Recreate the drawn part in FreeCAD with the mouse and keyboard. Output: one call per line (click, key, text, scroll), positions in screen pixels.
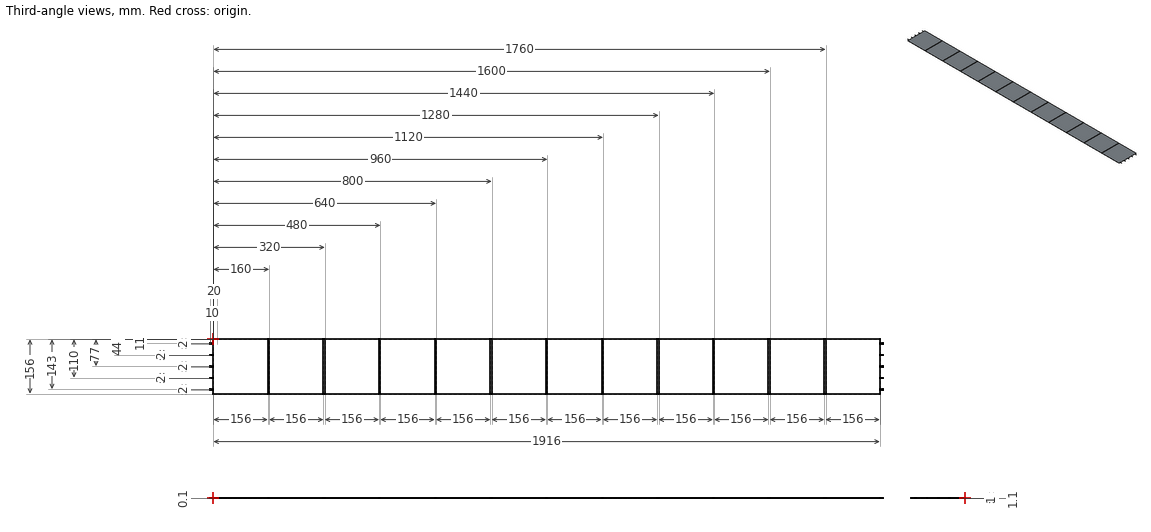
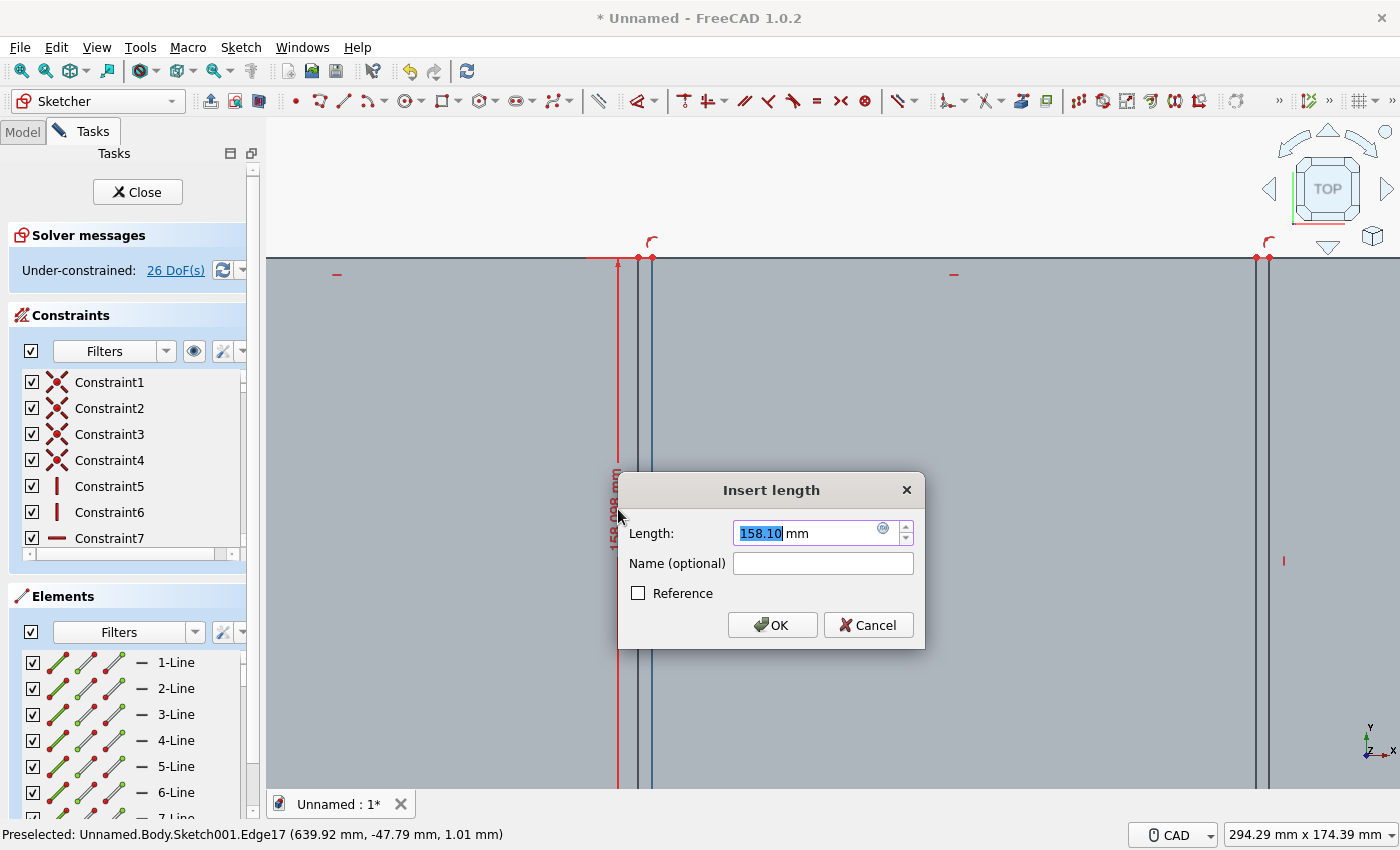
text(156)
key(Return)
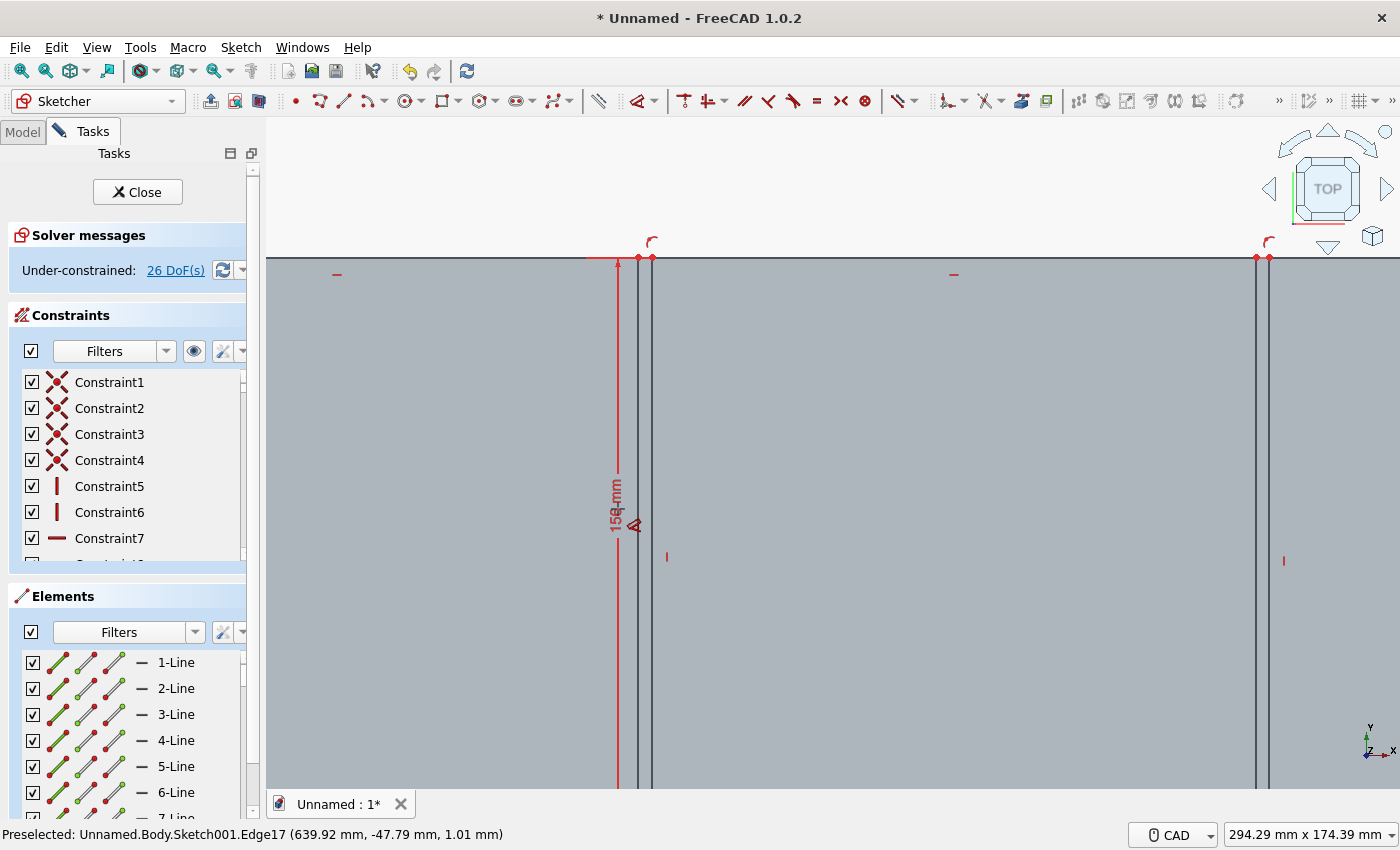
scroll(653, 442, down, 12)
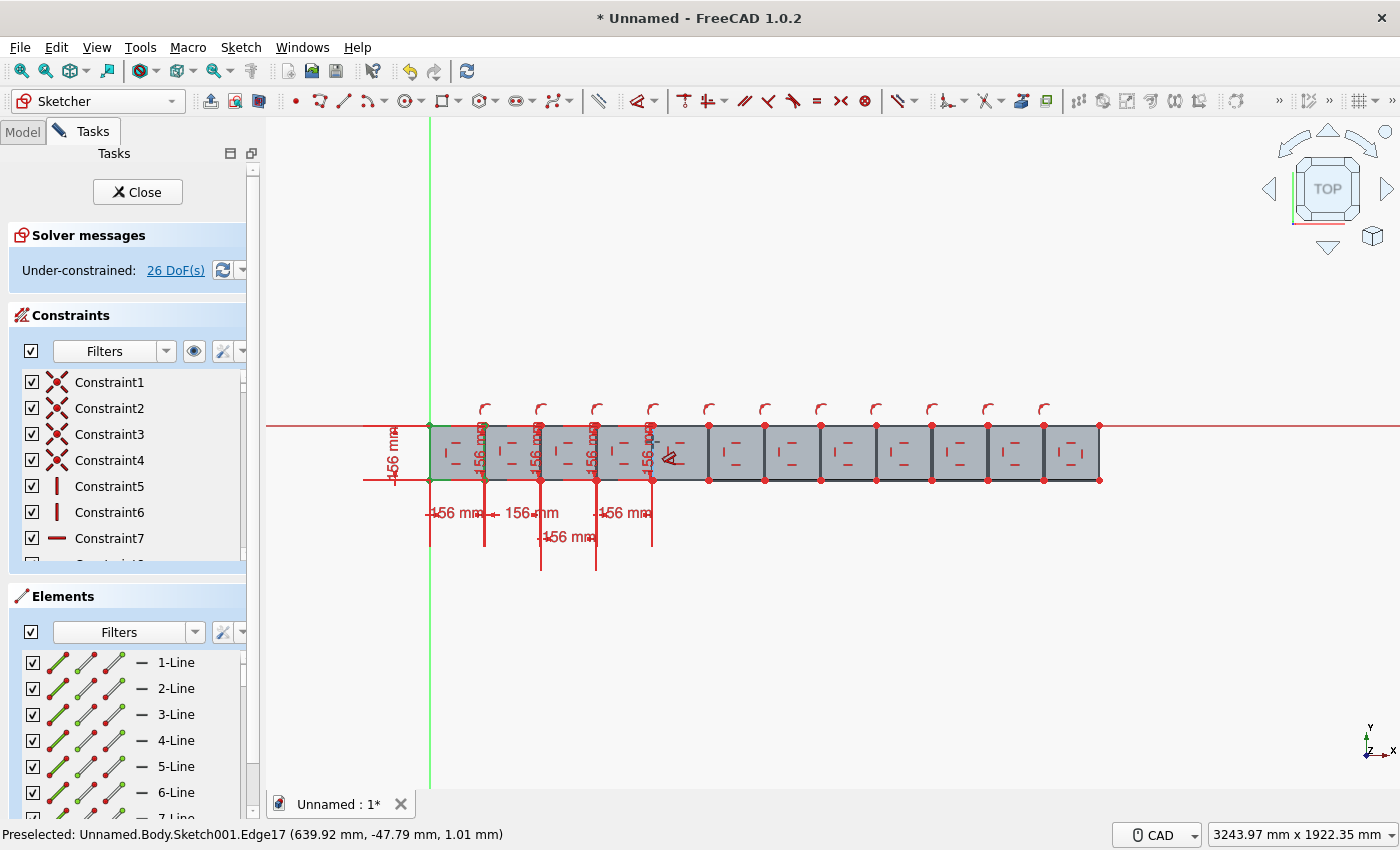
click(670, 480)
click(700, 514)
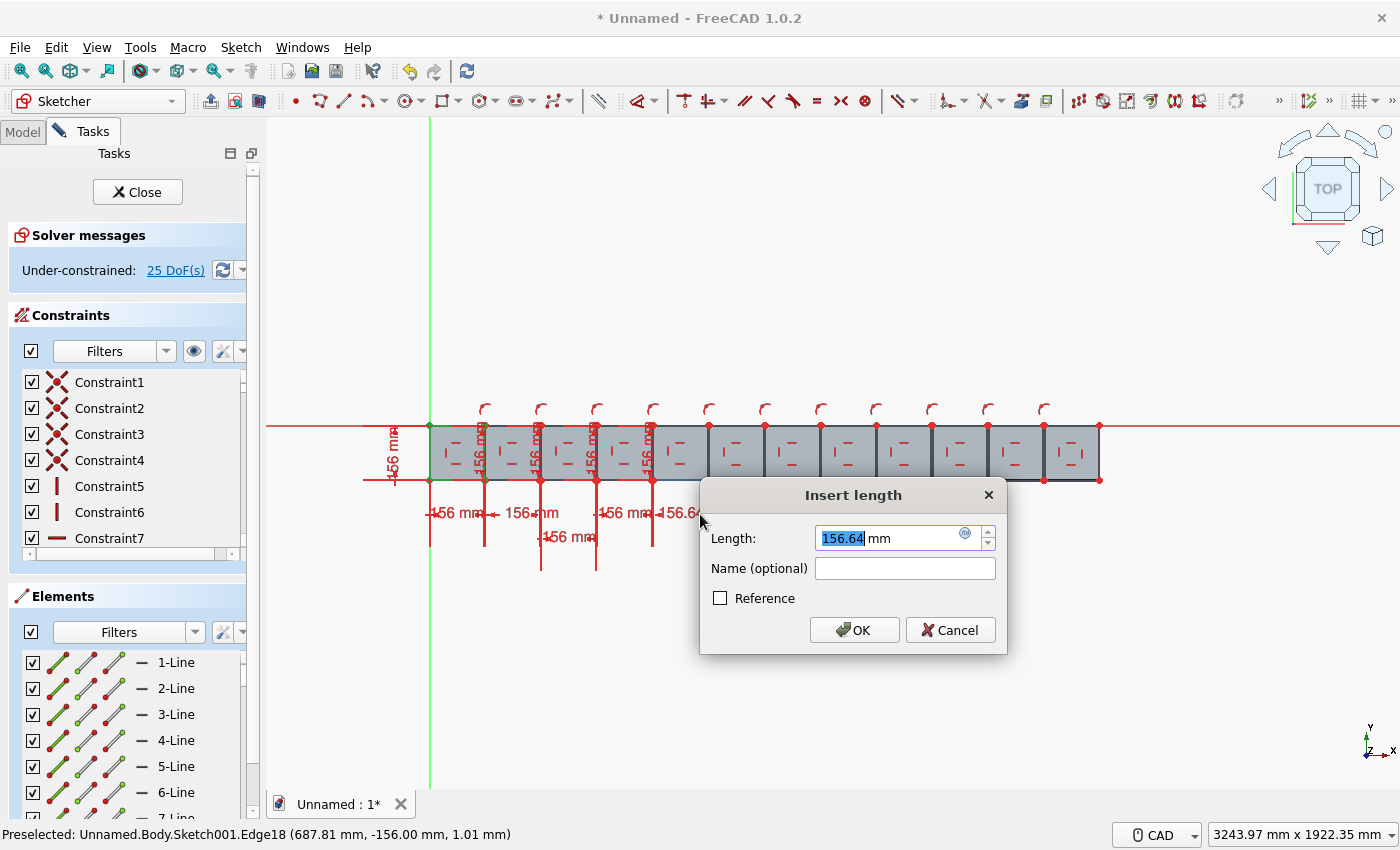
text(156)
key(Return)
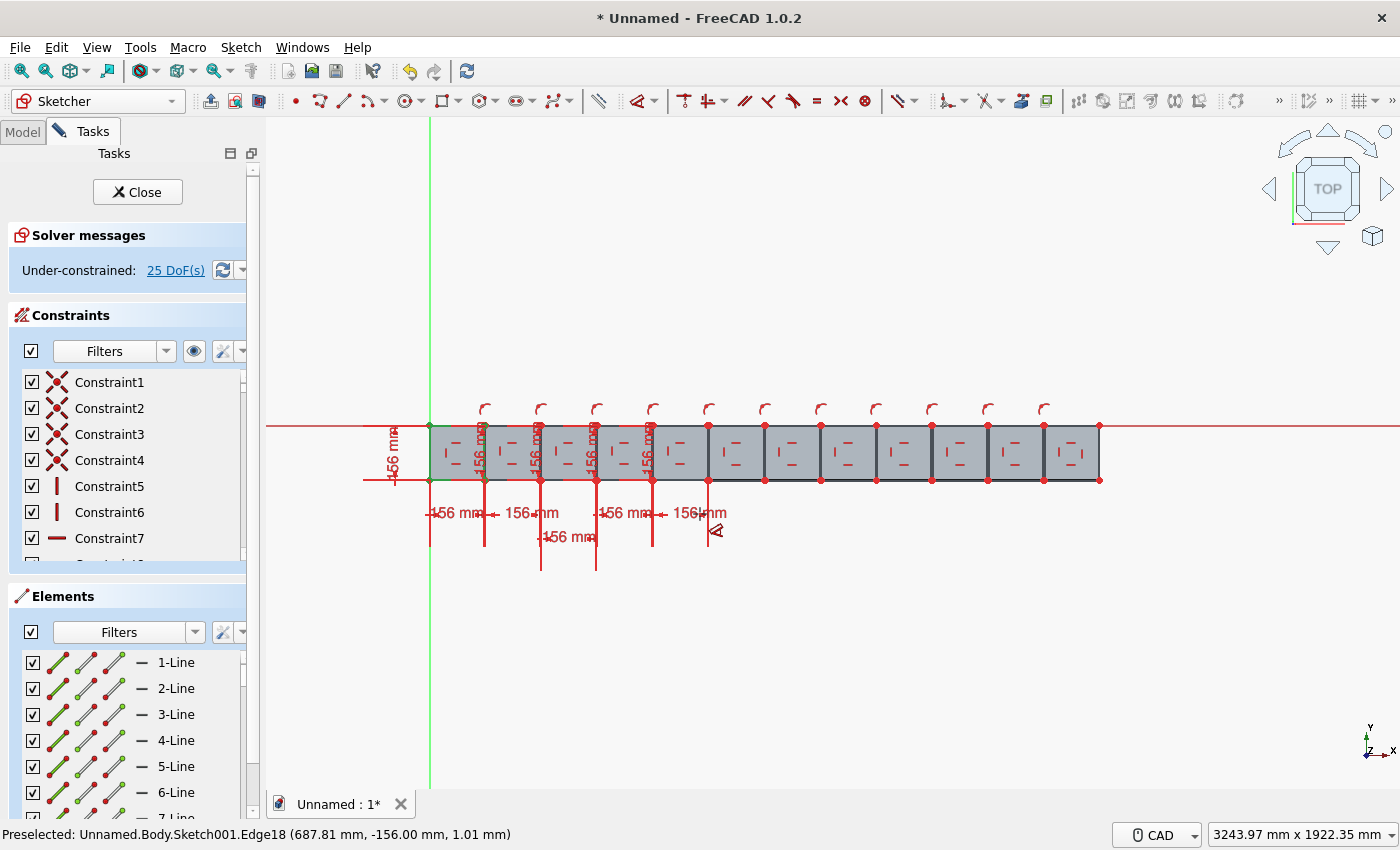
scroll(709, 442, up, 12)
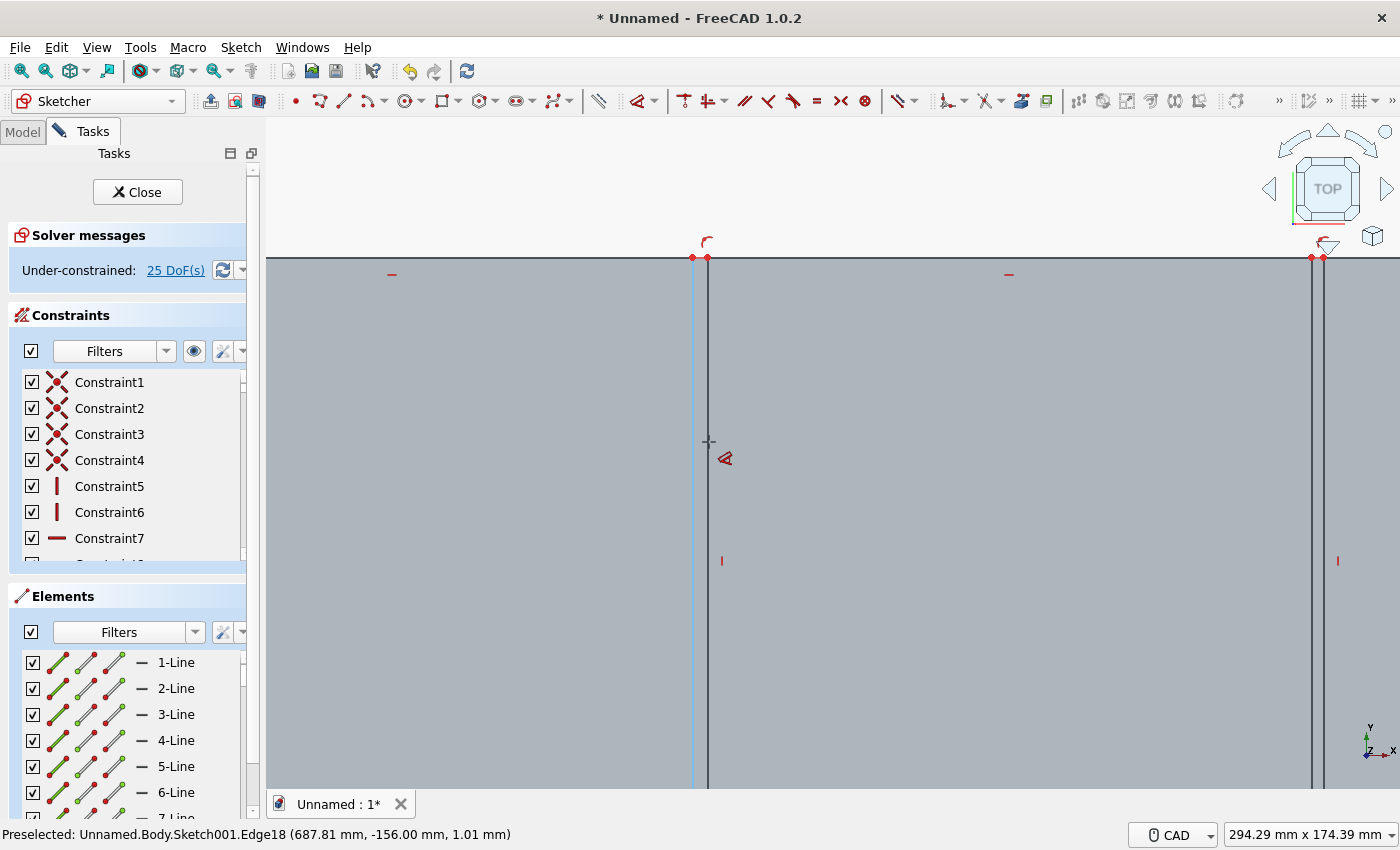
click(708, 441)
click(674, 509)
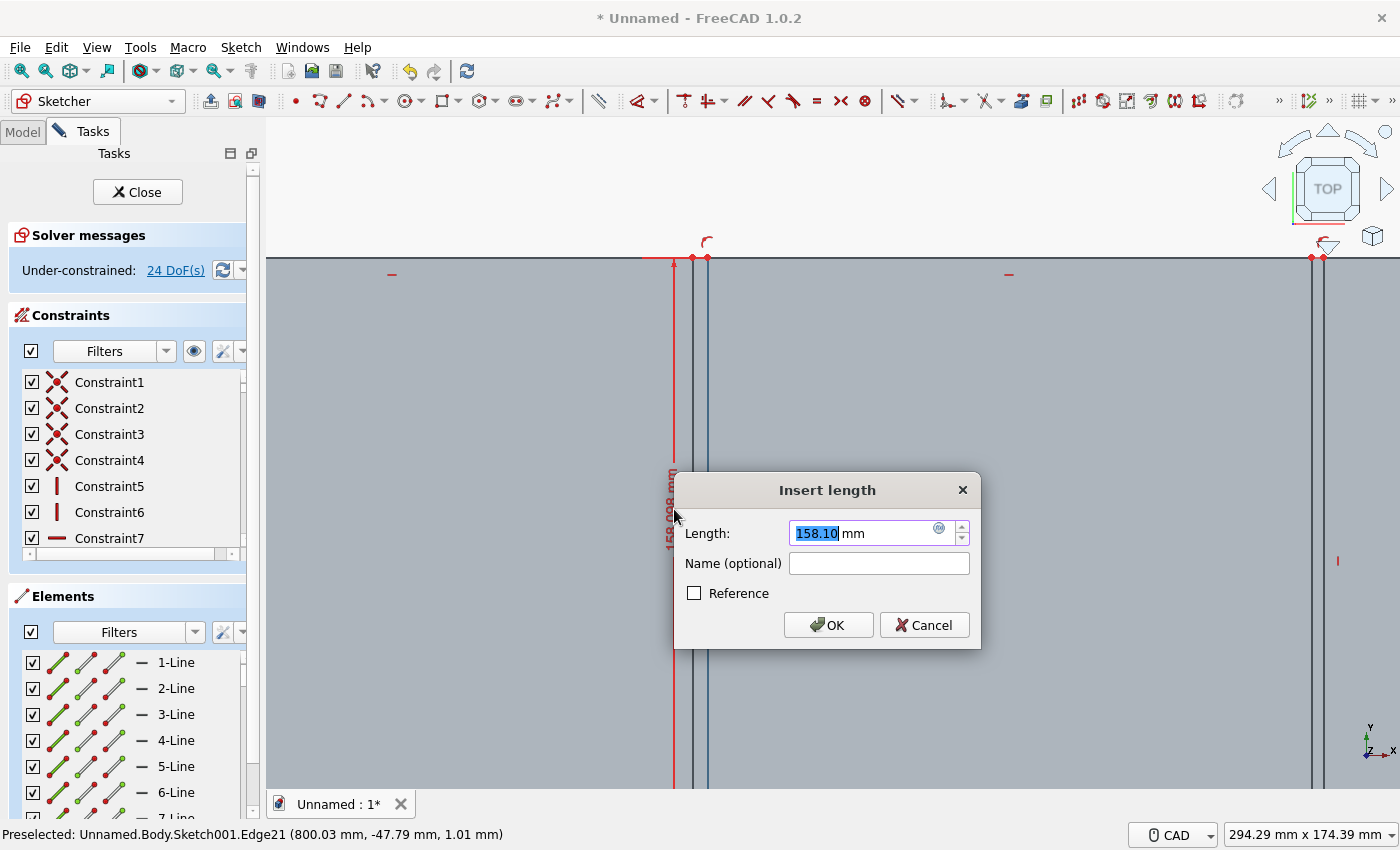
text(156)
key(Return)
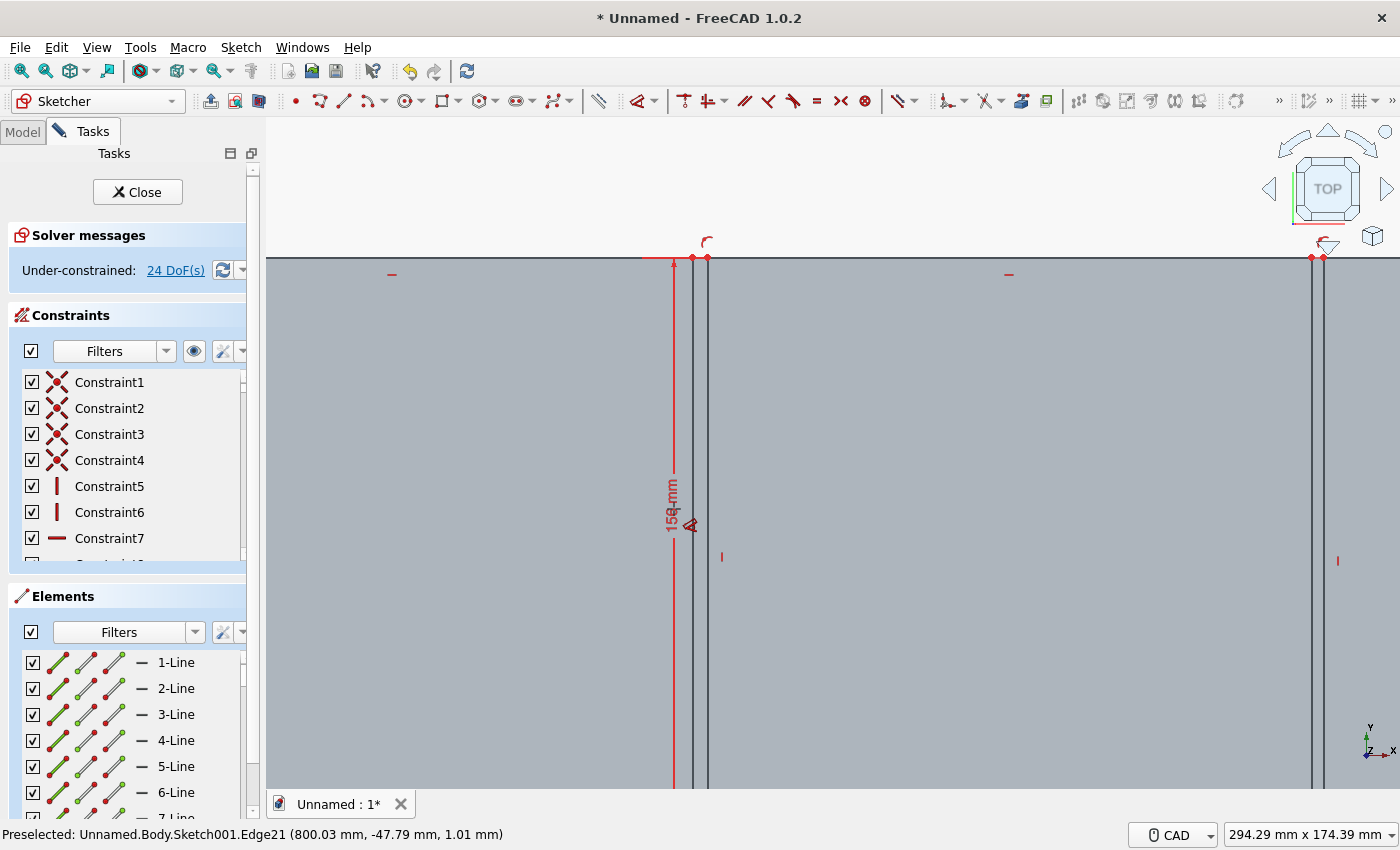
scroll(709, 442, down, 12)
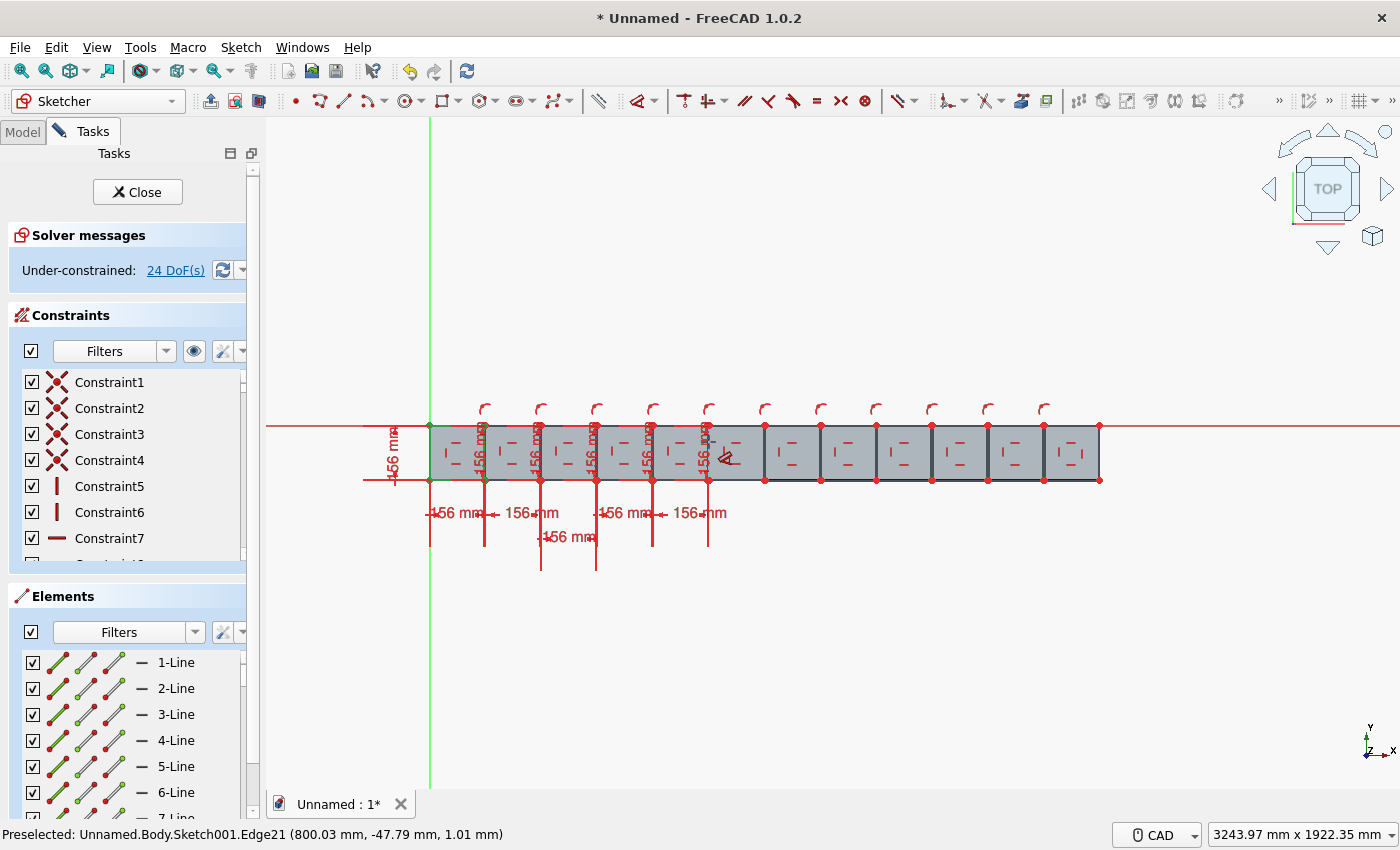
click(726, 480)
click(737, 538)